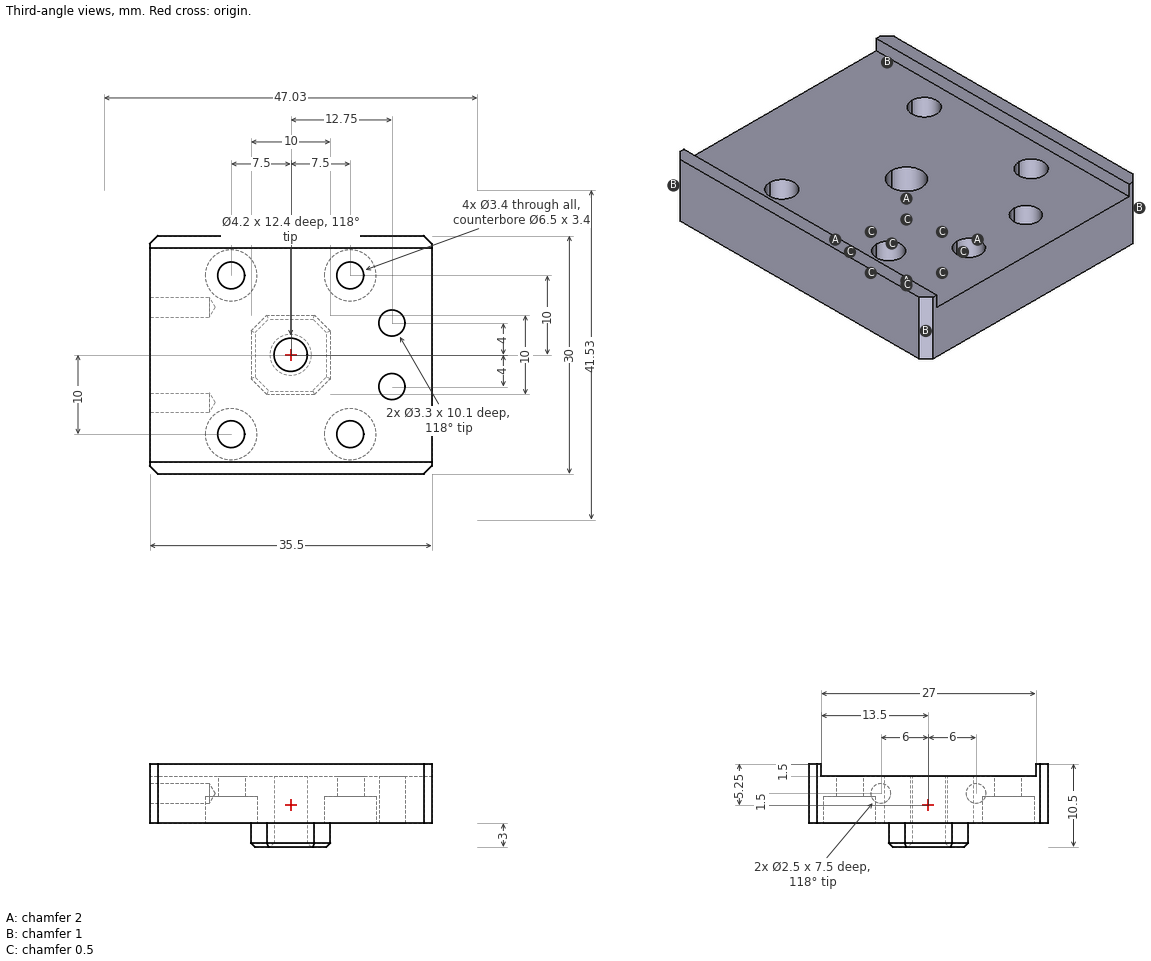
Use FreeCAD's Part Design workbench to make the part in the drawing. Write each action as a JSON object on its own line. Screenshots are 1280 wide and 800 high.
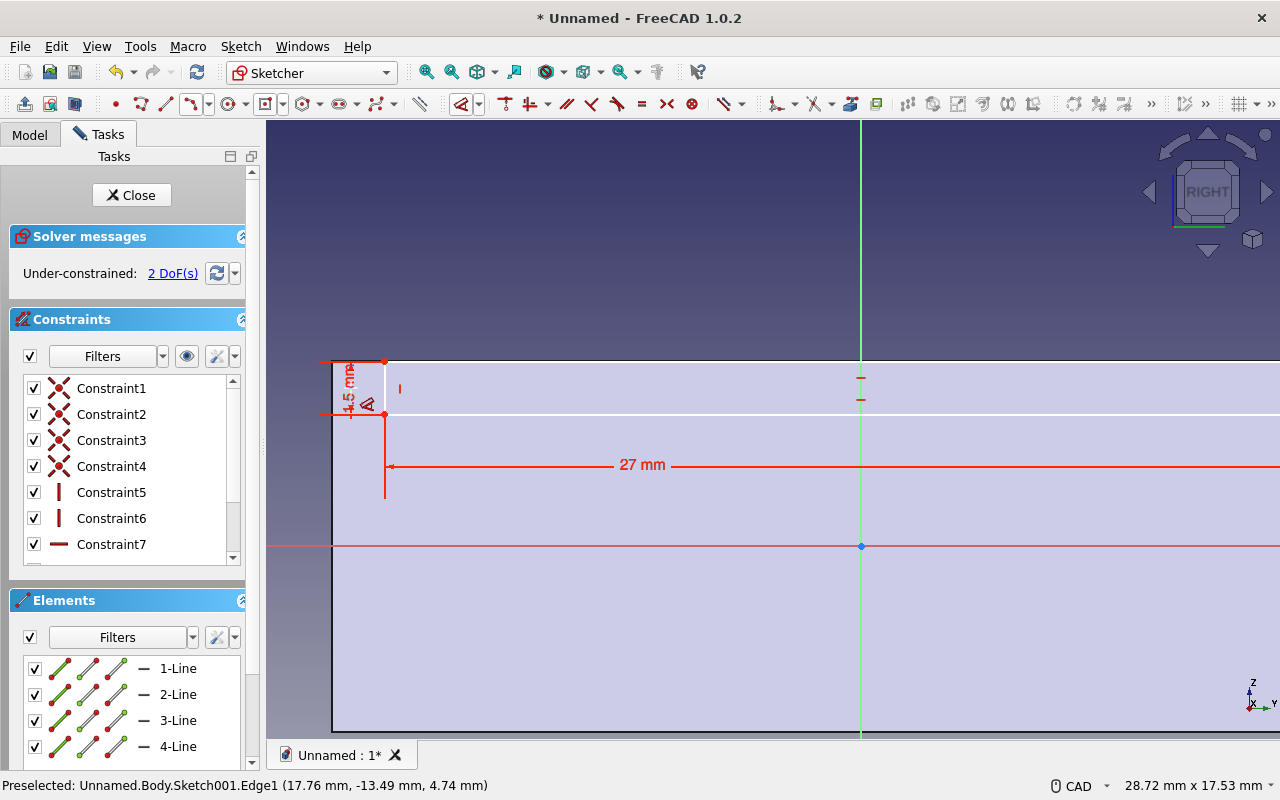
{"action": "left_click", "coordinate": [385, 362]}
{"action": "left_click", "coordinate": [623, 580]}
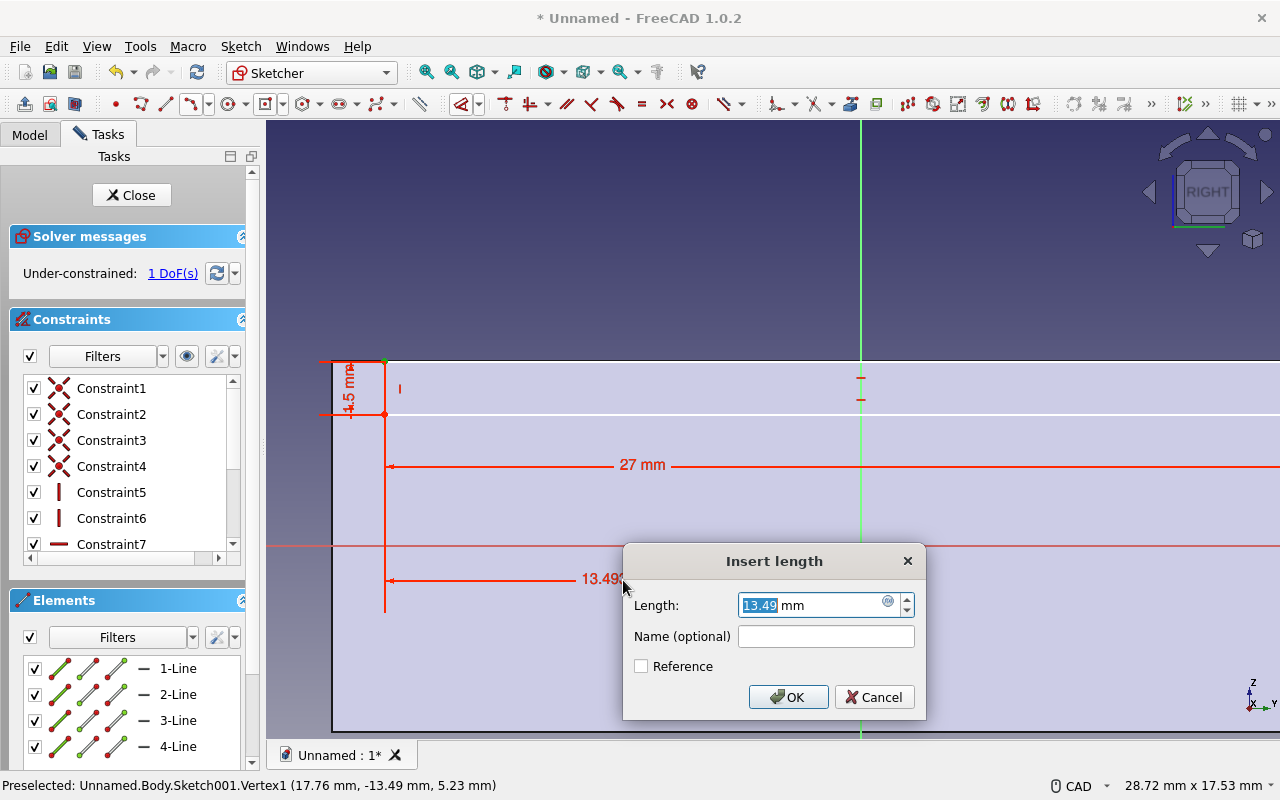
{"action": "type", "text": "13.5"}
{"action": "key", "text": "Return"}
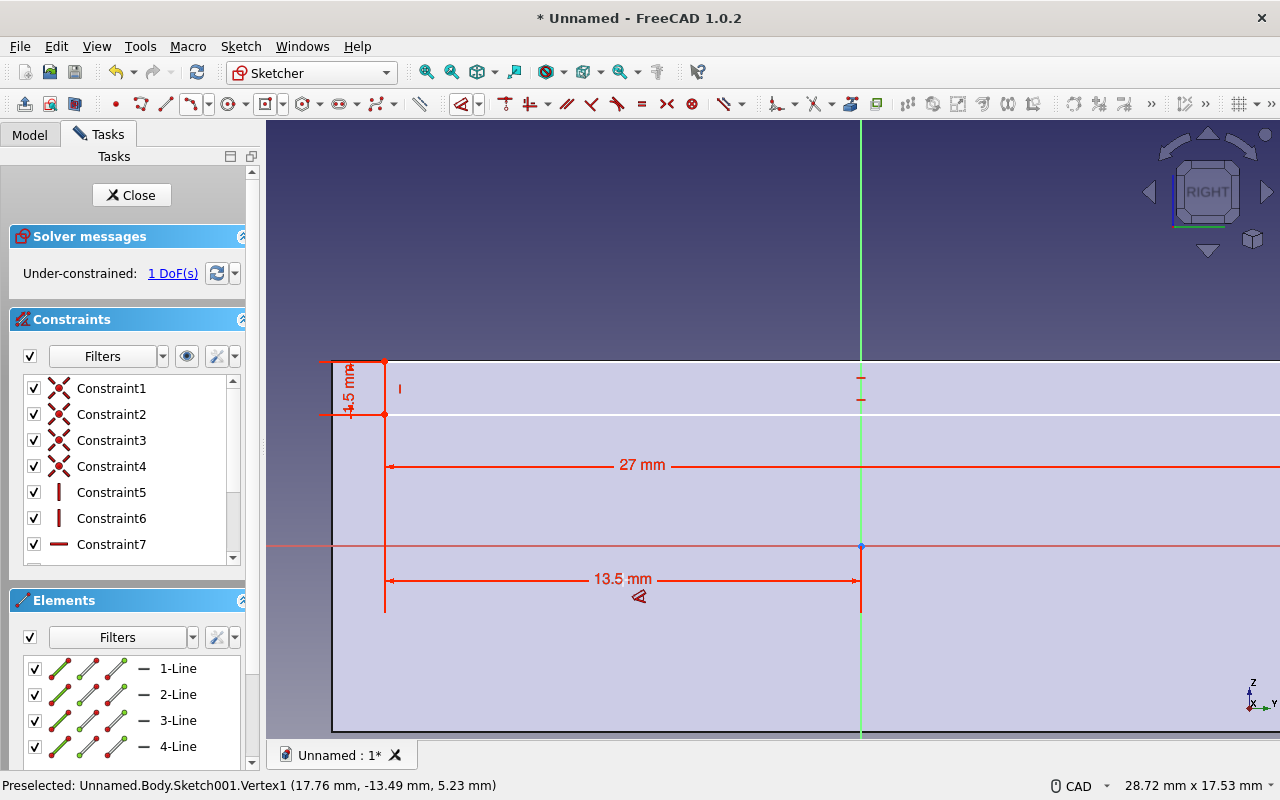
{"action": "left_click", "coordinate": [385, 362]}
{"action": "left_click", "coordinate": [351, 454]}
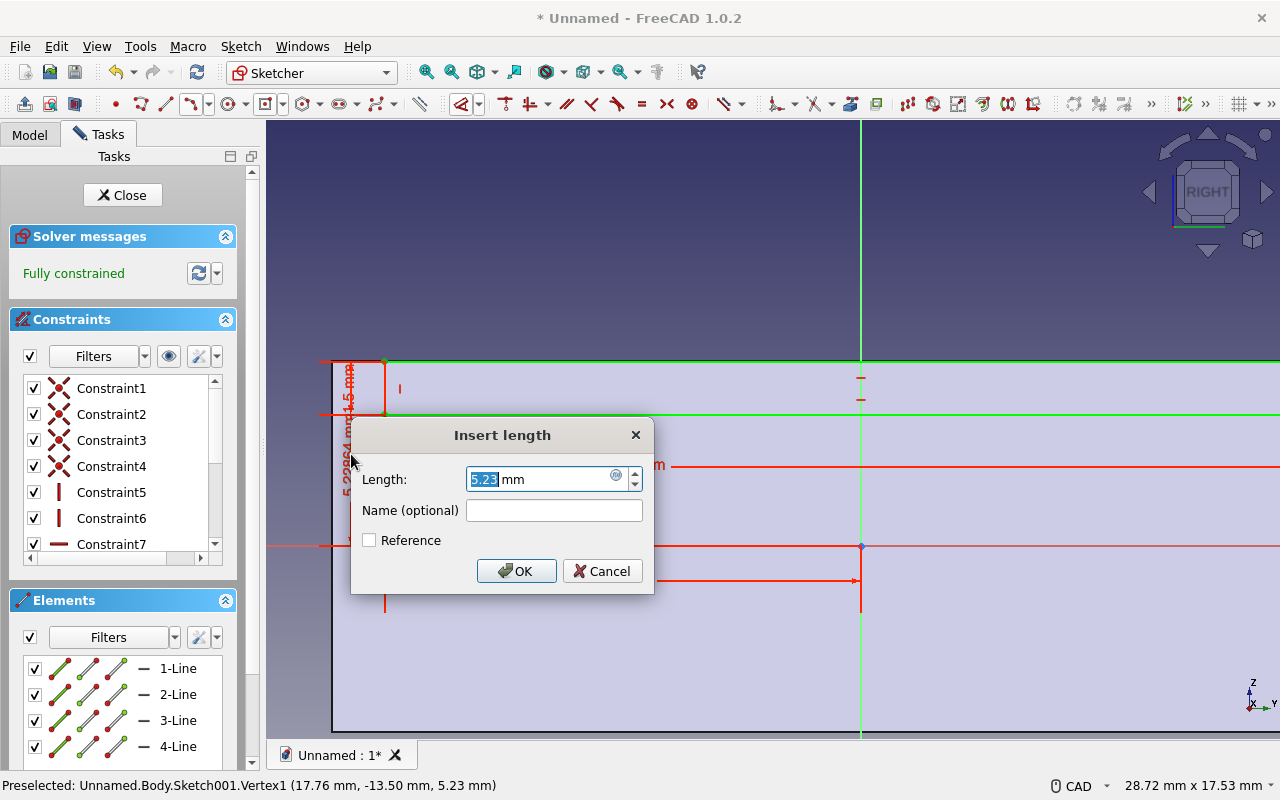
{"action": "type", "text": "5.25"}
{"action": "key", "text": "Return"}
{"action": "key", "text": "Escape"}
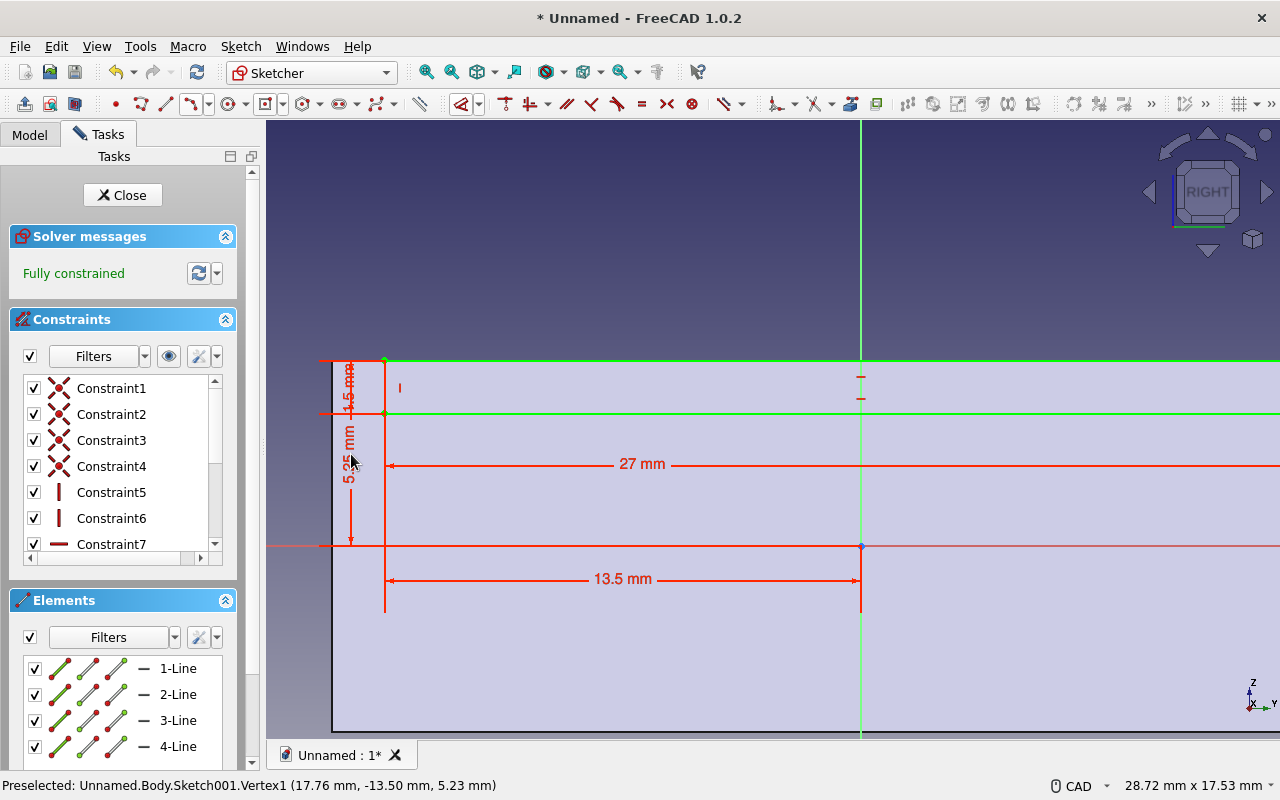
{"action": "left_click", "coordinate": [123, 195]}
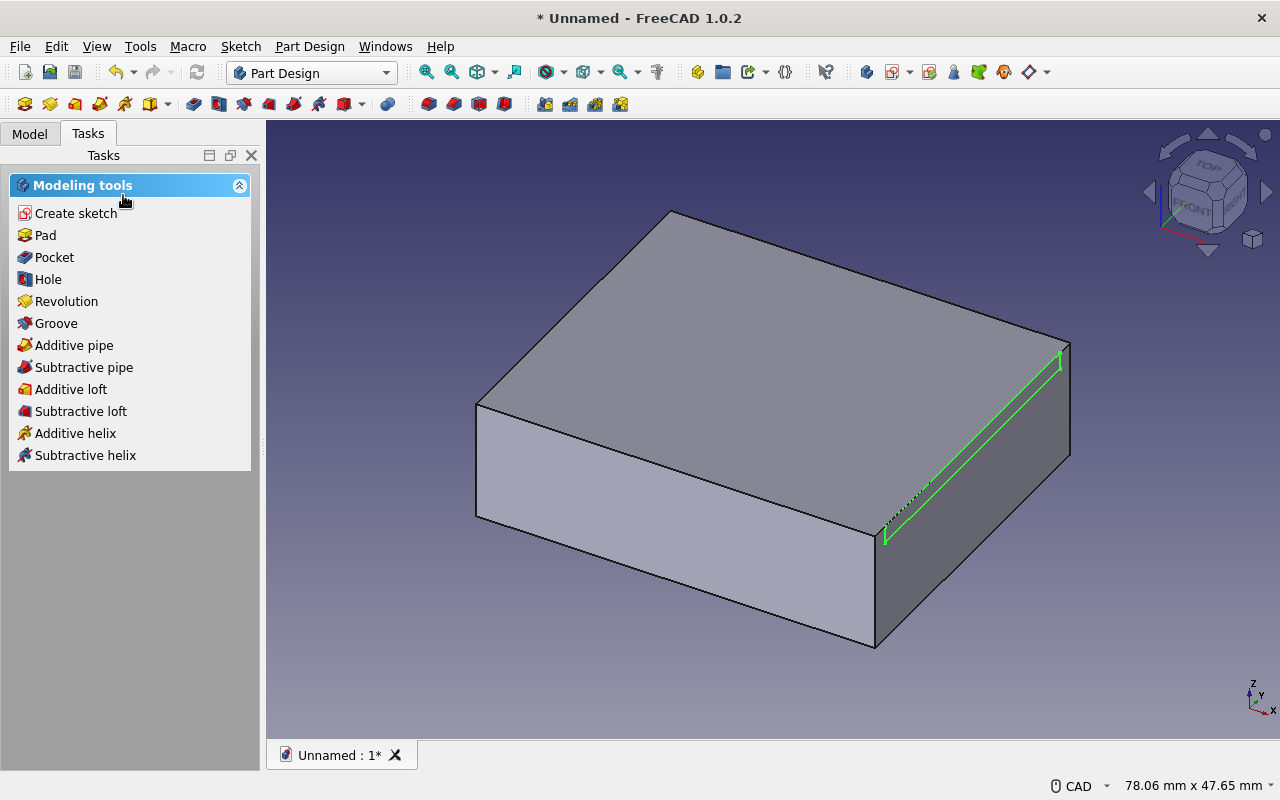
{"action": "left_click", "coordinate": [194, 104]}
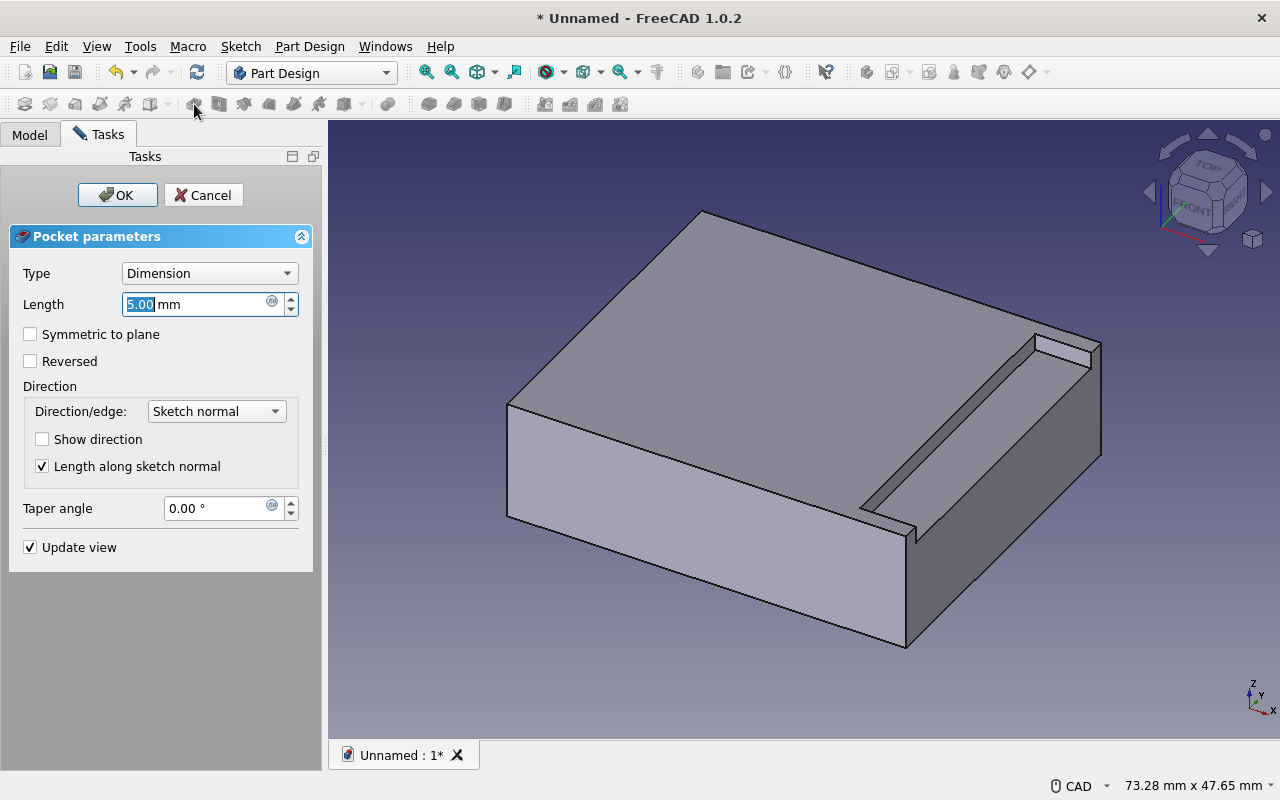
{"action": "left_click", "coordinate": [210, 274]}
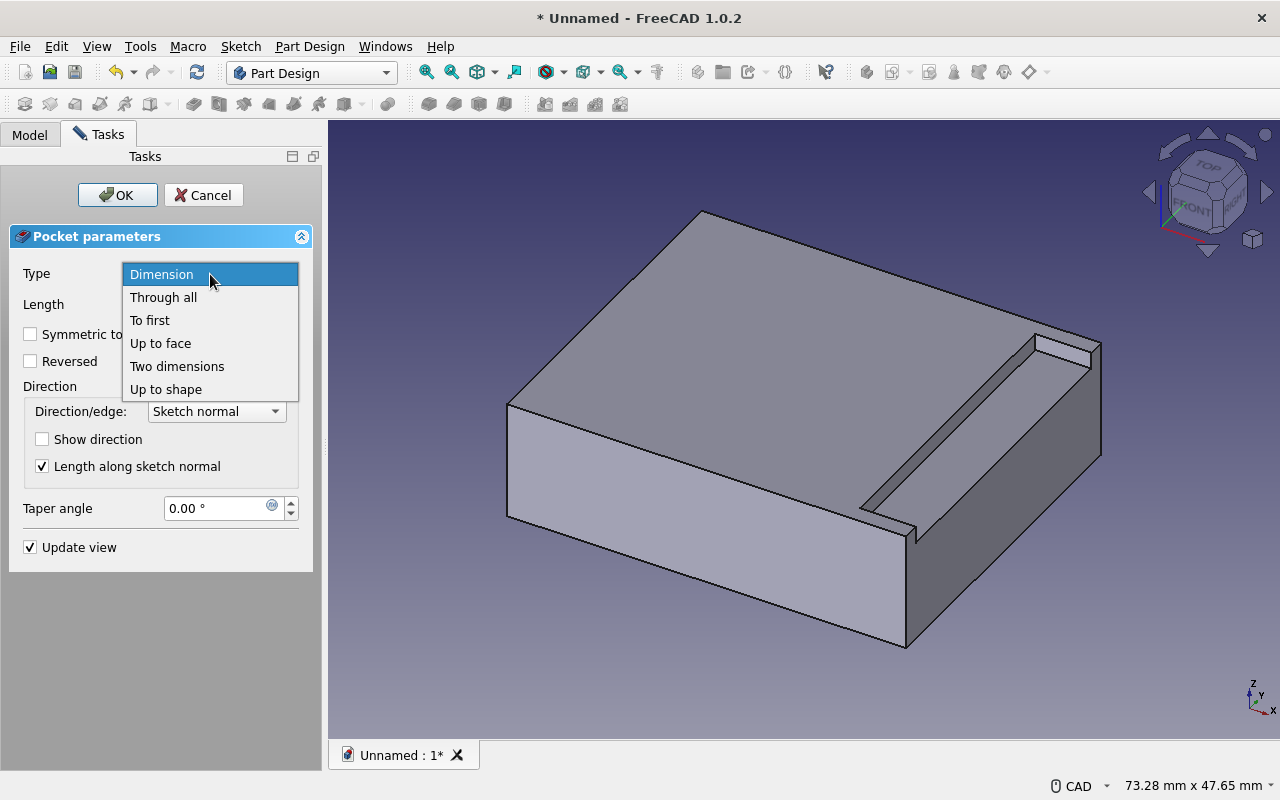
{"action": "left_click", "coordinate": [208, 298]}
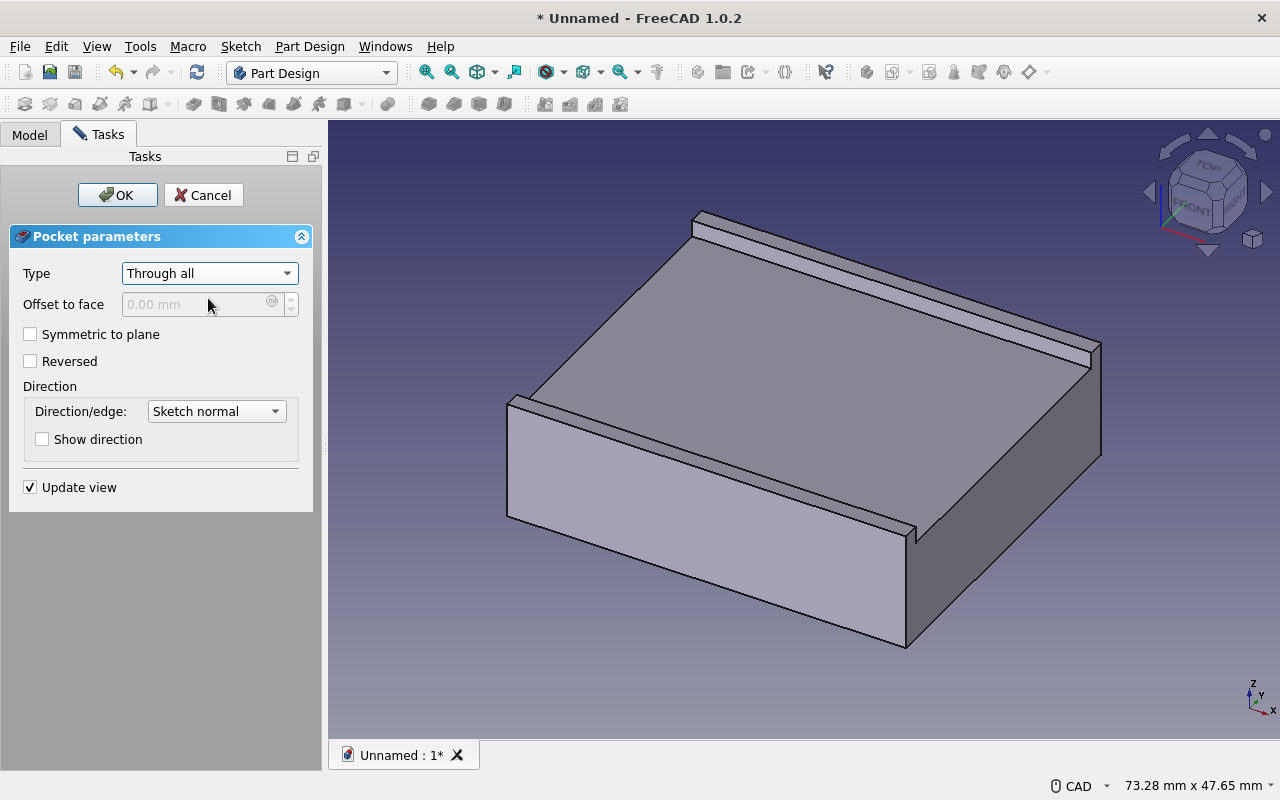
{"action": "left_click", "coordinate": [118, 195]}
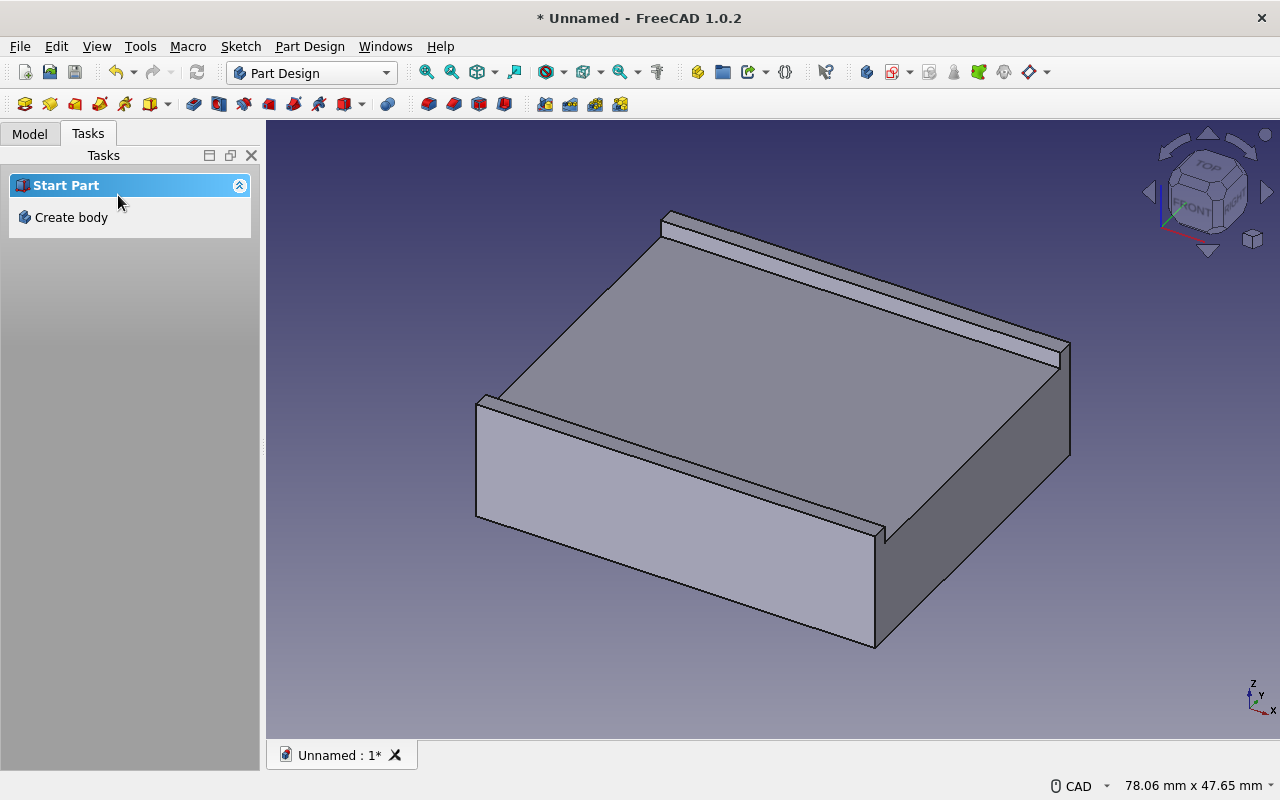
{"action": "key", "text": "5"}